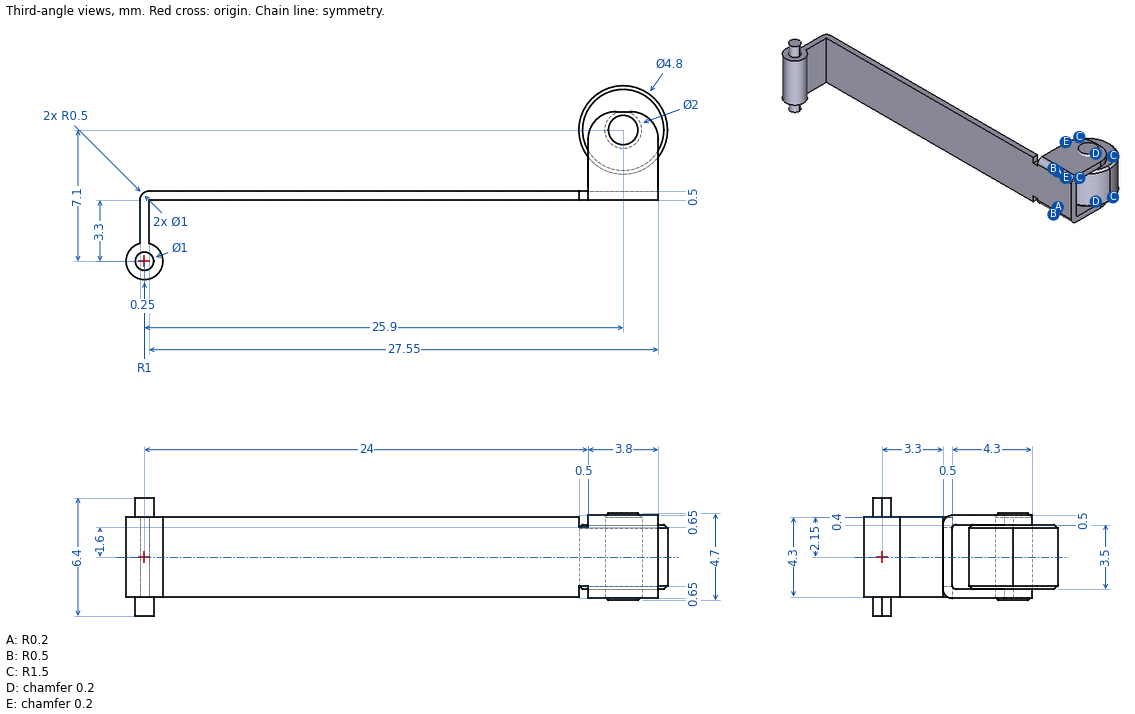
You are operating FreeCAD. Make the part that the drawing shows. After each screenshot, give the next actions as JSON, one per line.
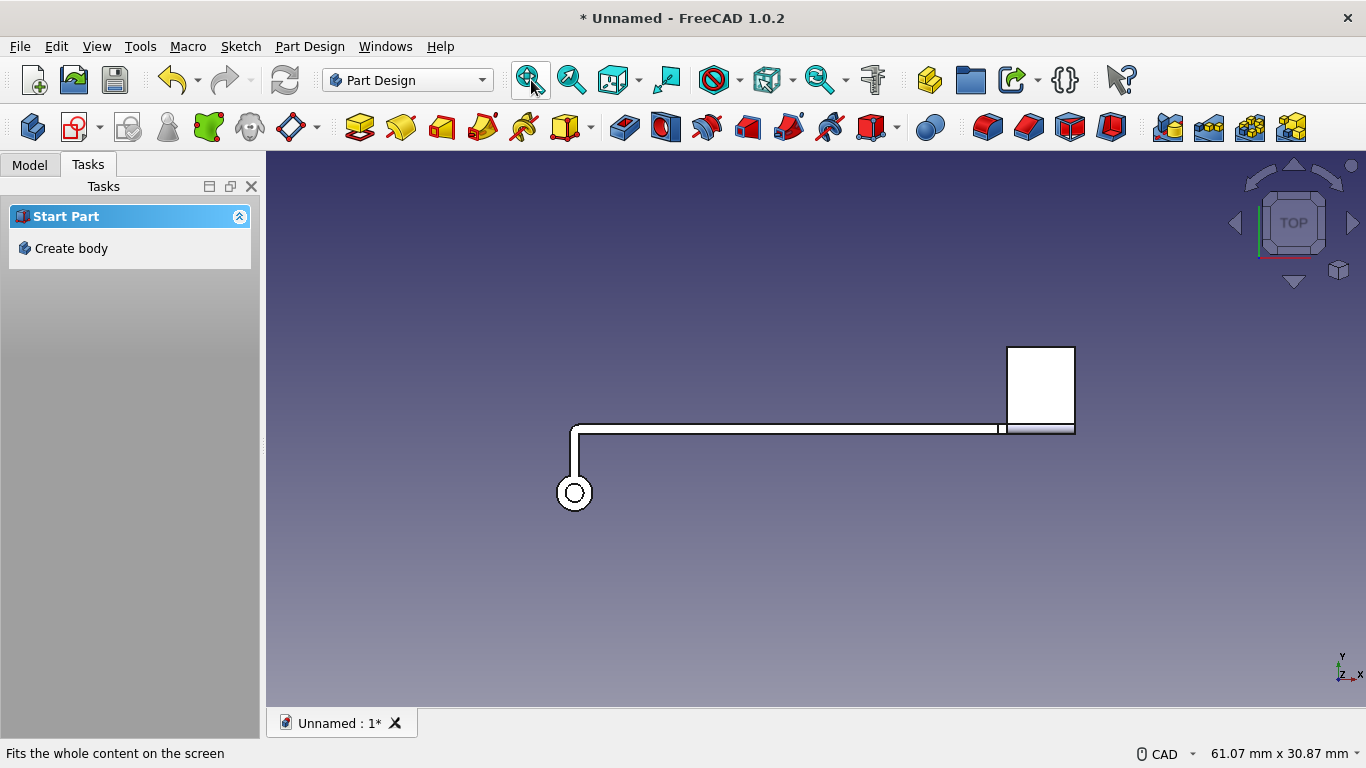
{"action": "scroll", "coordinate": [1007, 346], "scroll_direction": "up", "scroll_amount": 8}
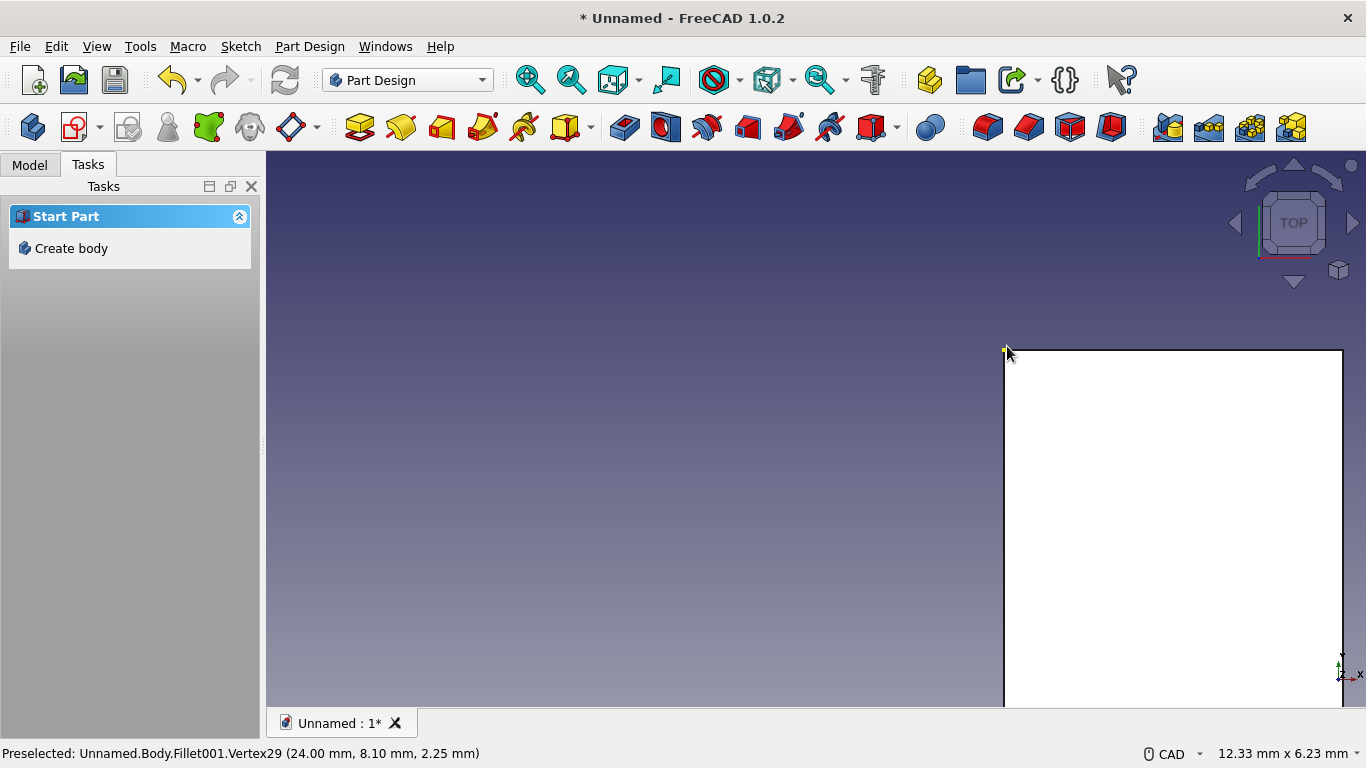
{"action": "left_click", "coordinate": [531, 80]}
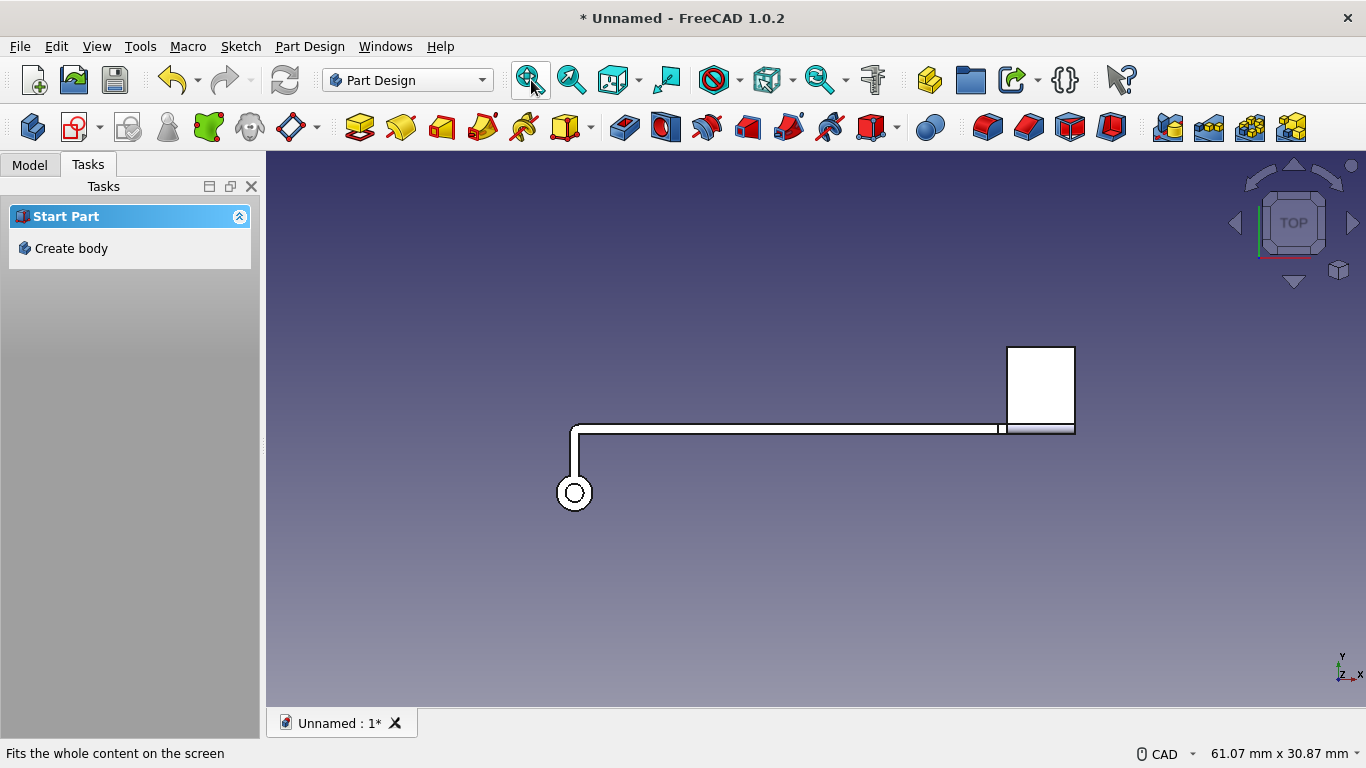
{"action": "key", "text": "1"}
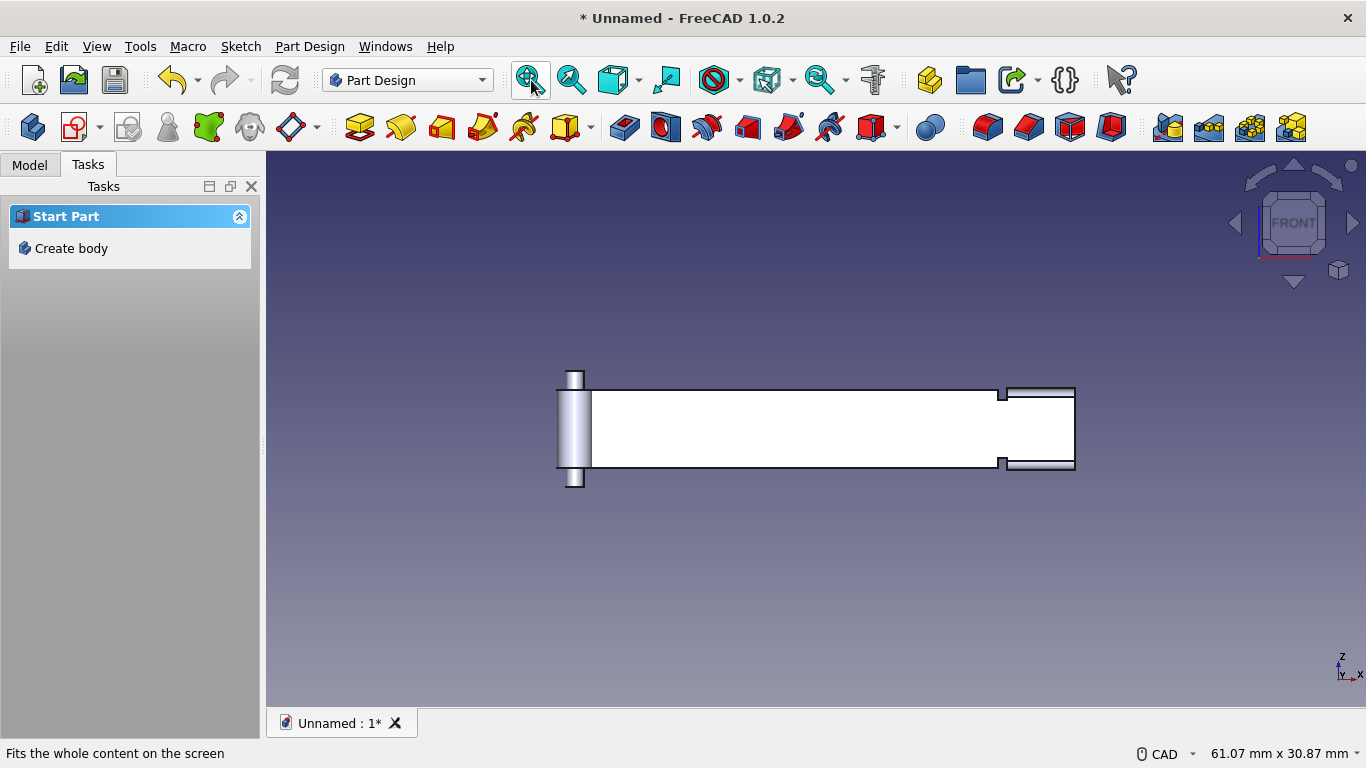
{"action": "scroll", "coordinate": [1007, 464], "scroll_direction": "up", "scroll_amount": 8}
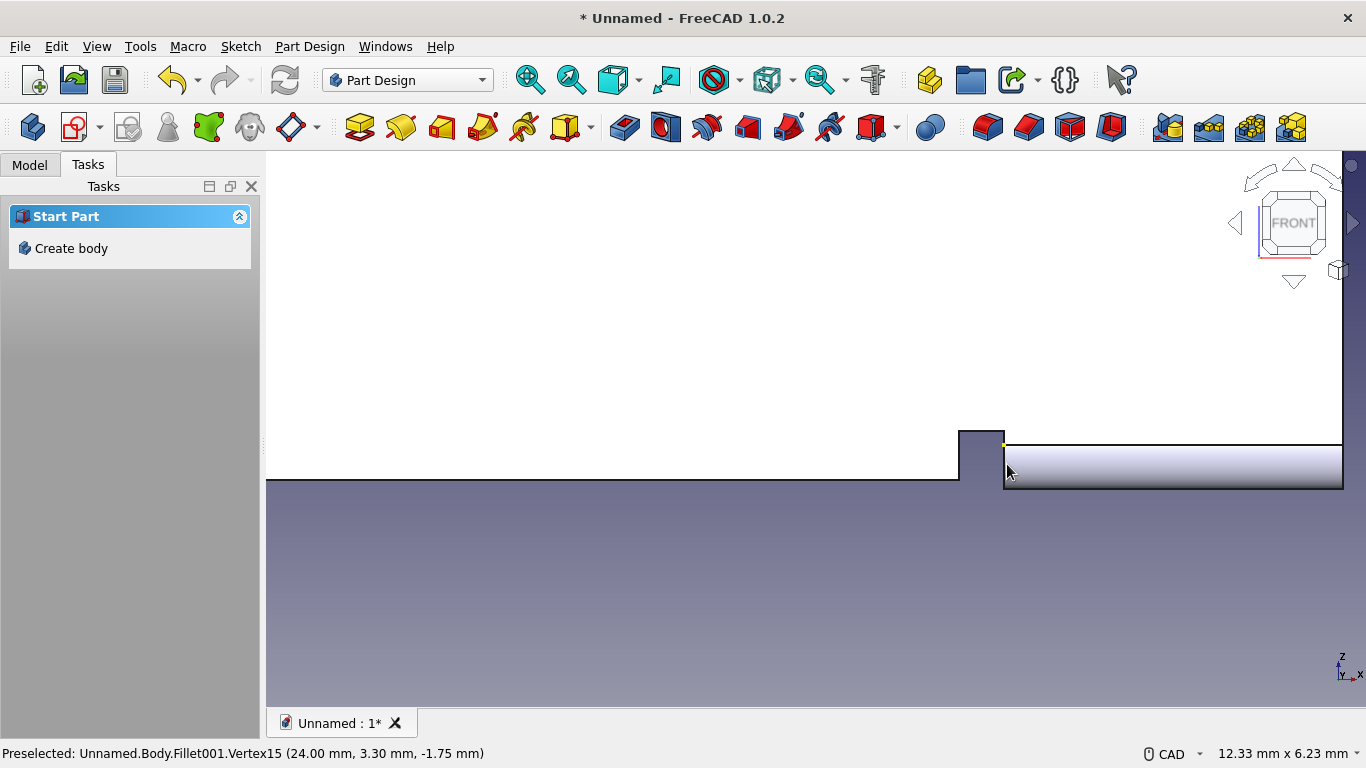
{"action": "left_click", "coordinate": [531, 80]}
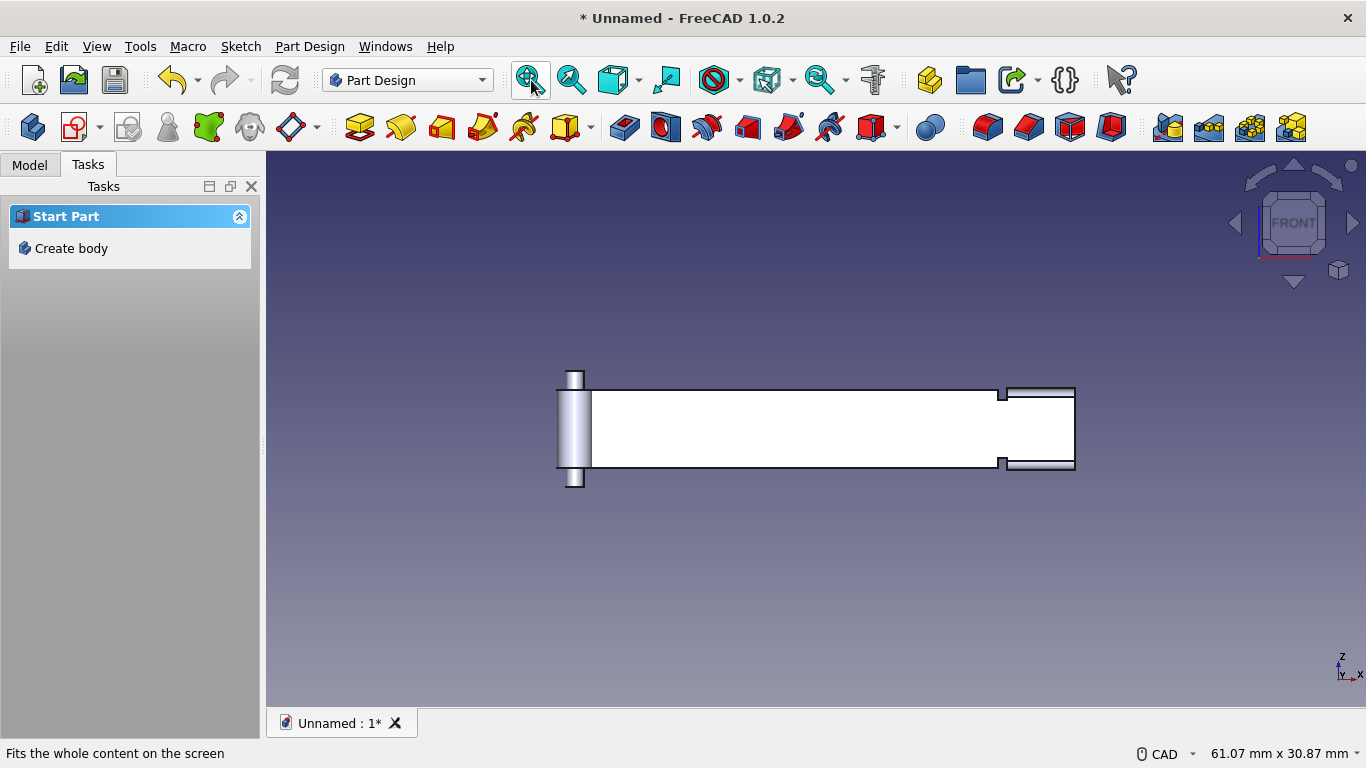
{"action": "key", "text": "3"}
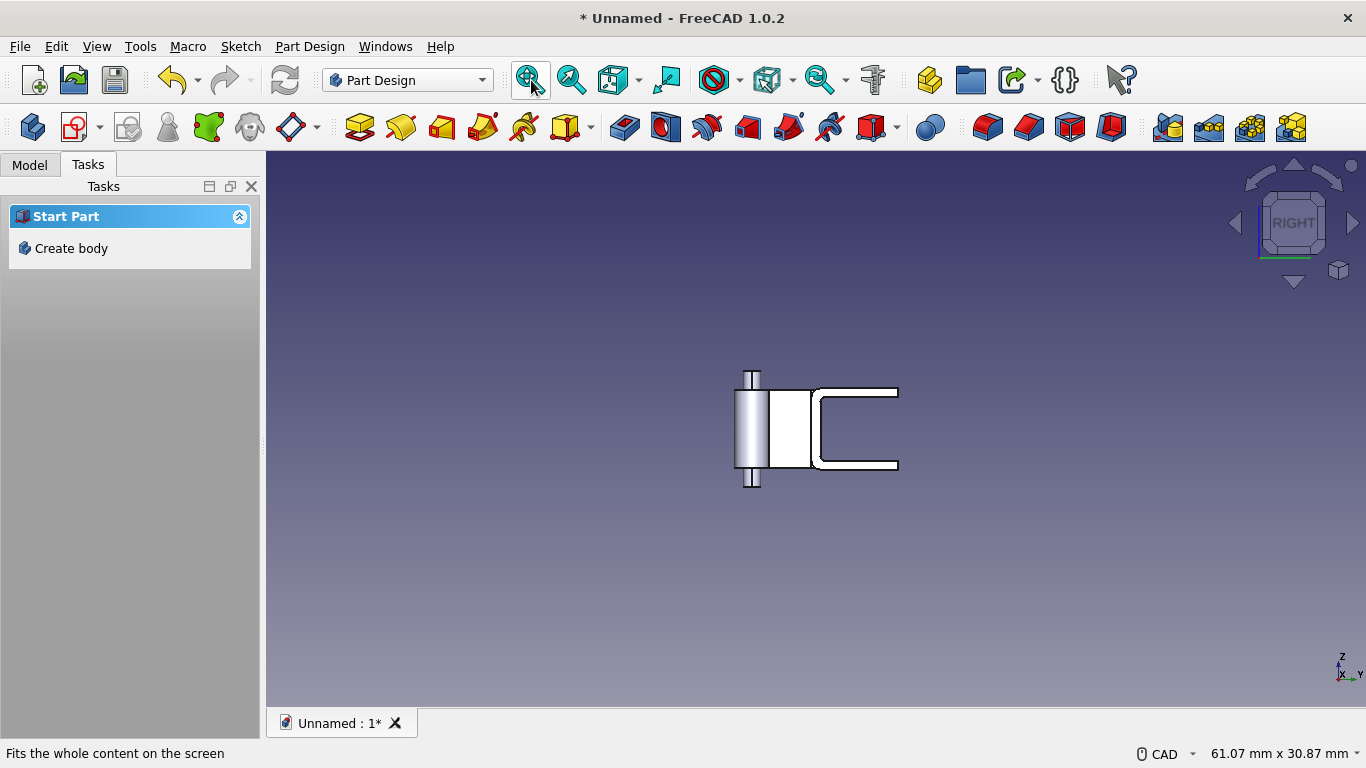
{"action": "key", "text": "v f"}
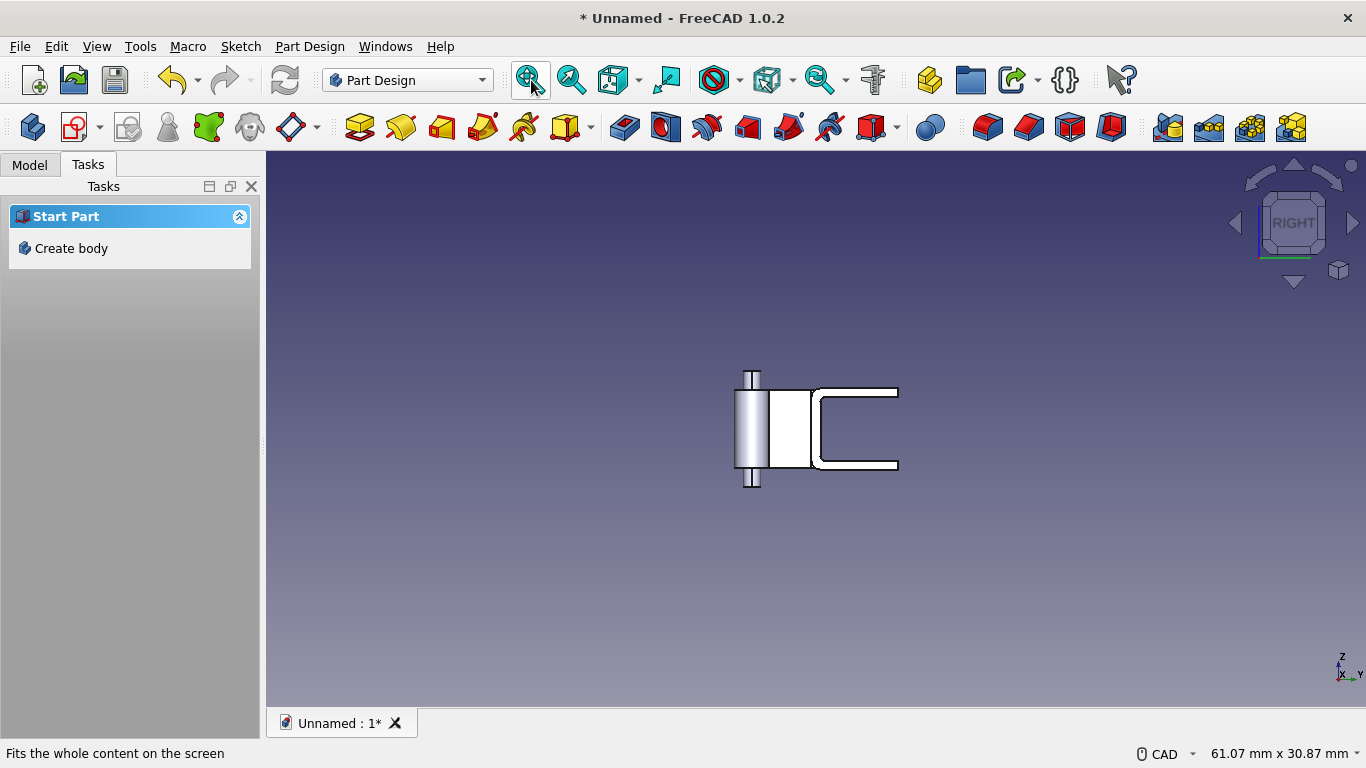
{"action": "scroll", "coordinate": [898, 464], "scroll_direction": "up", "scroll_amount": 8}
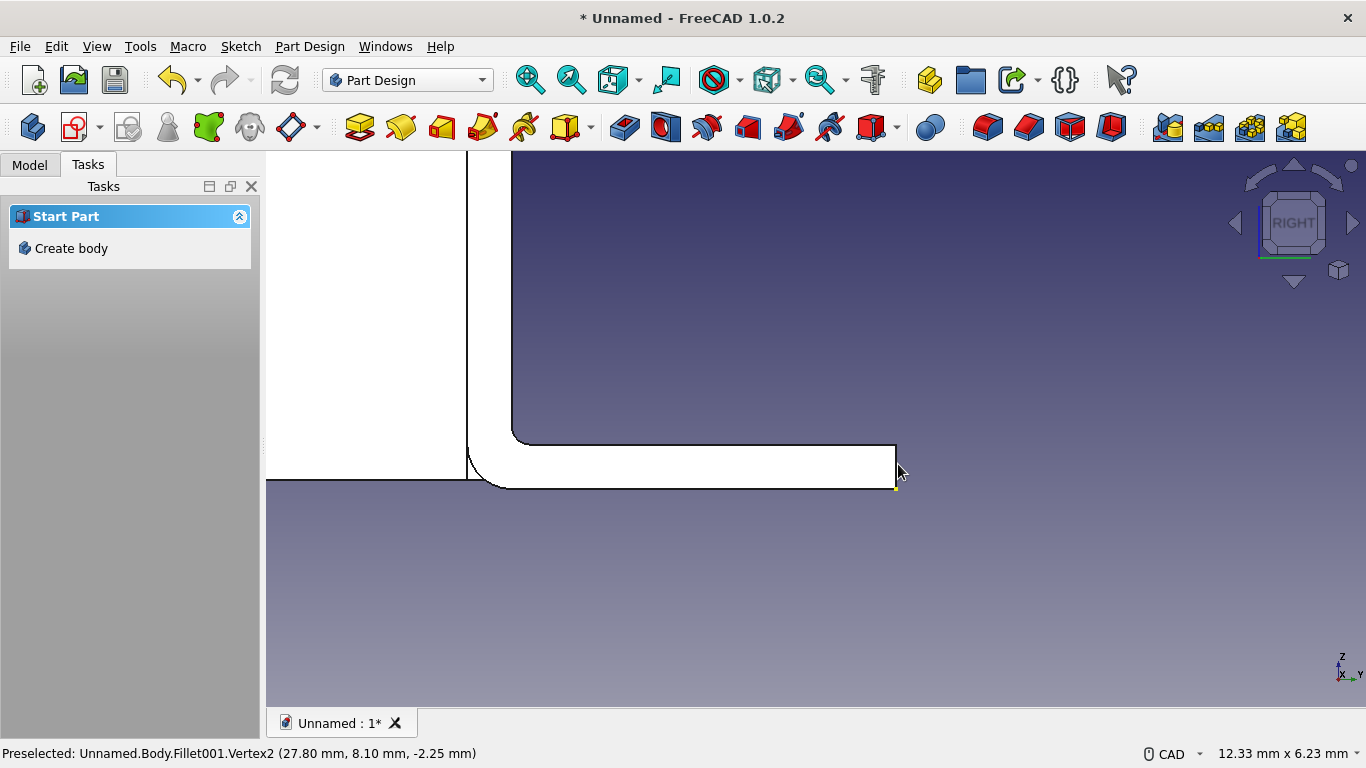
{"action": "left_click", "coordinate": [896, 466]}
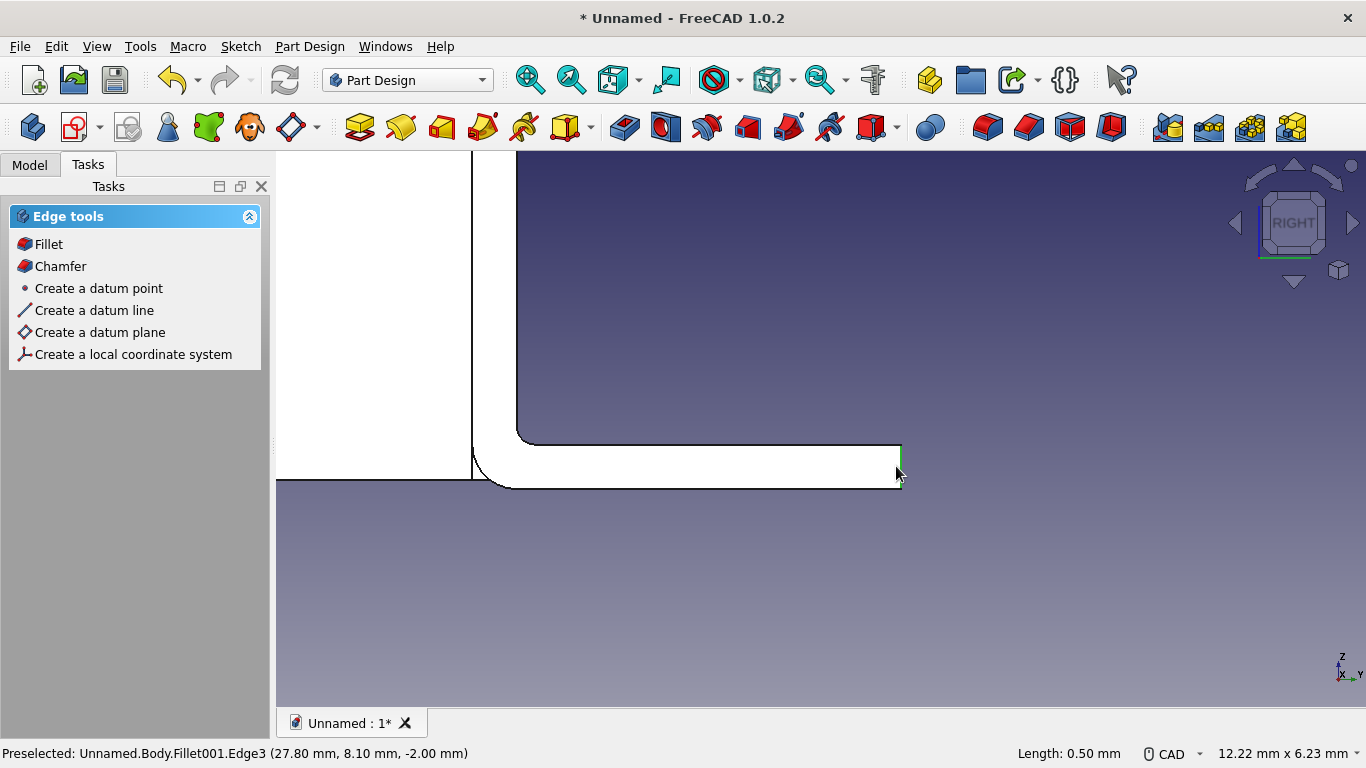
{"action": "key", "text": "v f"}